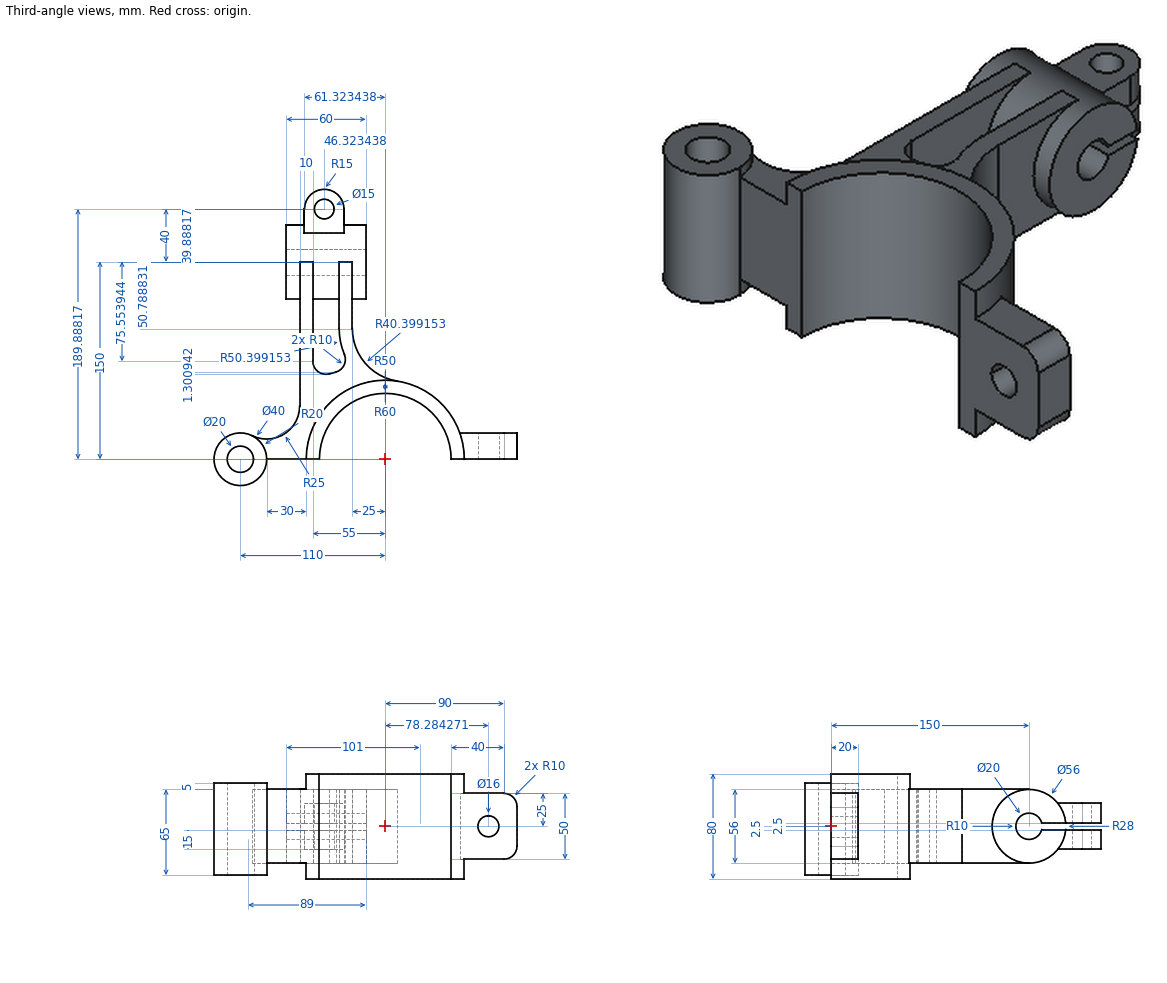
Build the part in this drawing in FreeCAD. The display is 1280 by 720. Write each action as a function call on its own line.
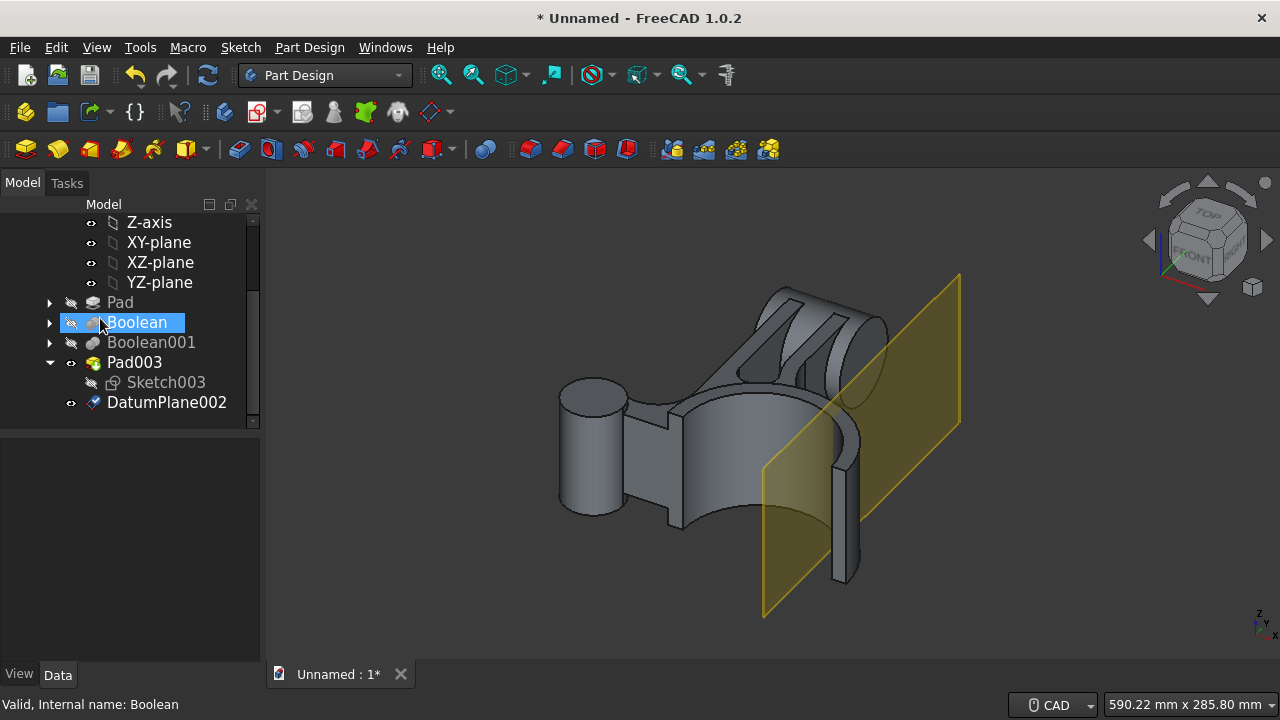
click(116, 403)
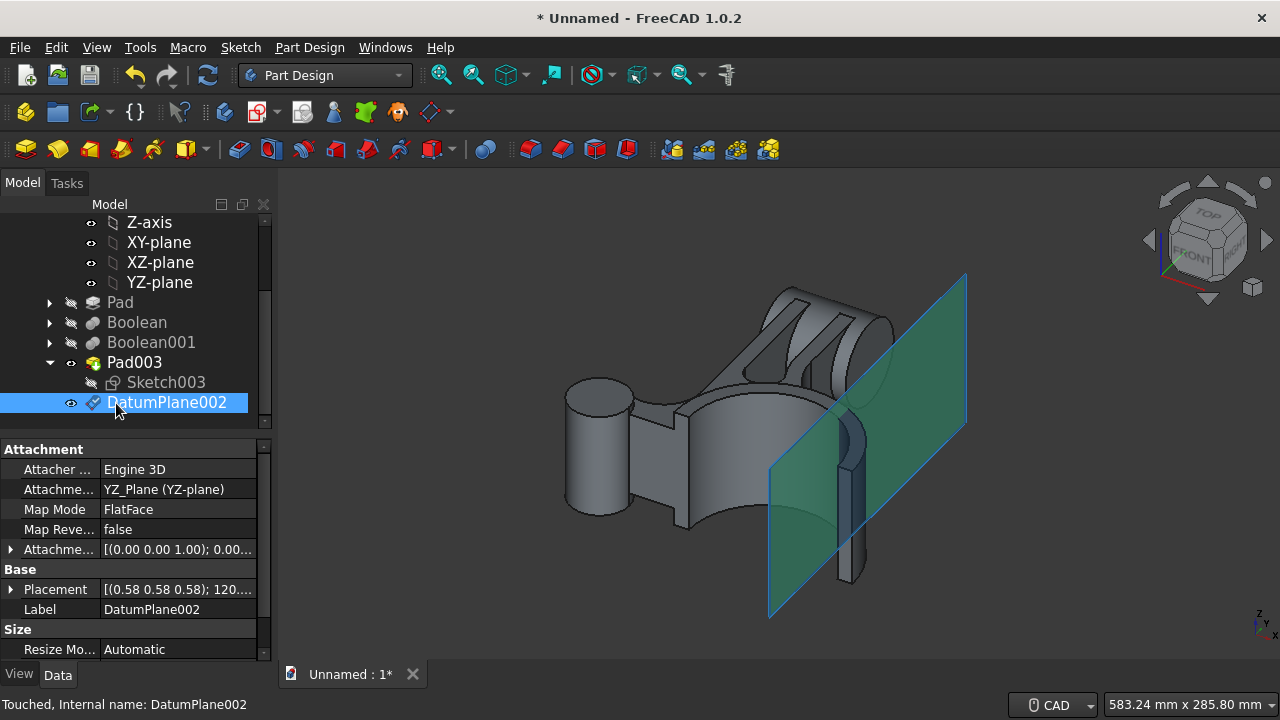
click(258, 112)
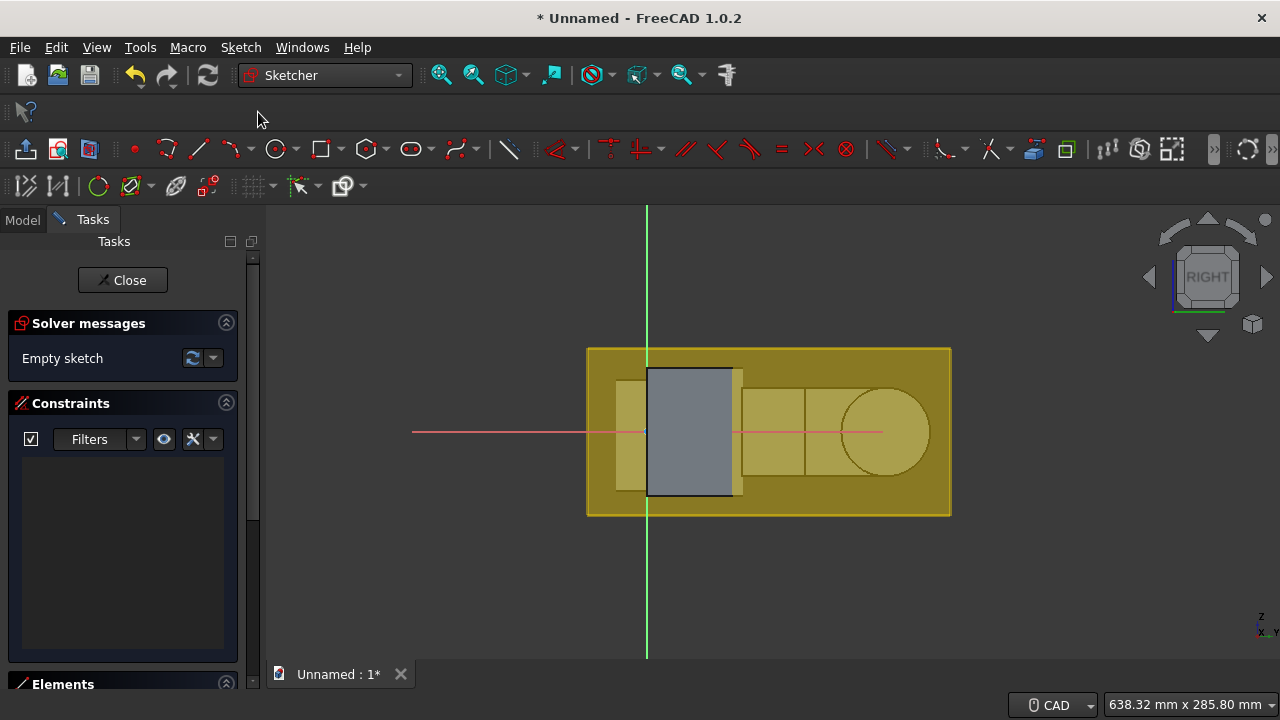
click(90, 150)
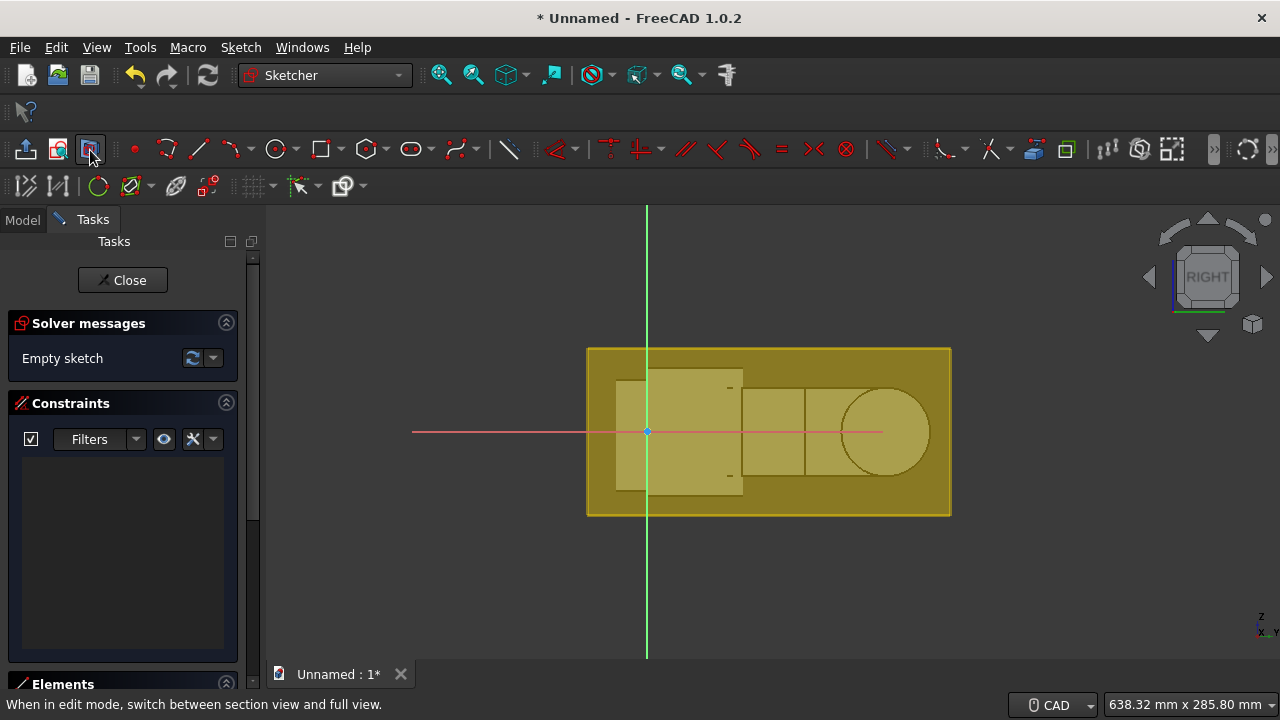
scroll(924, 432, up, 11)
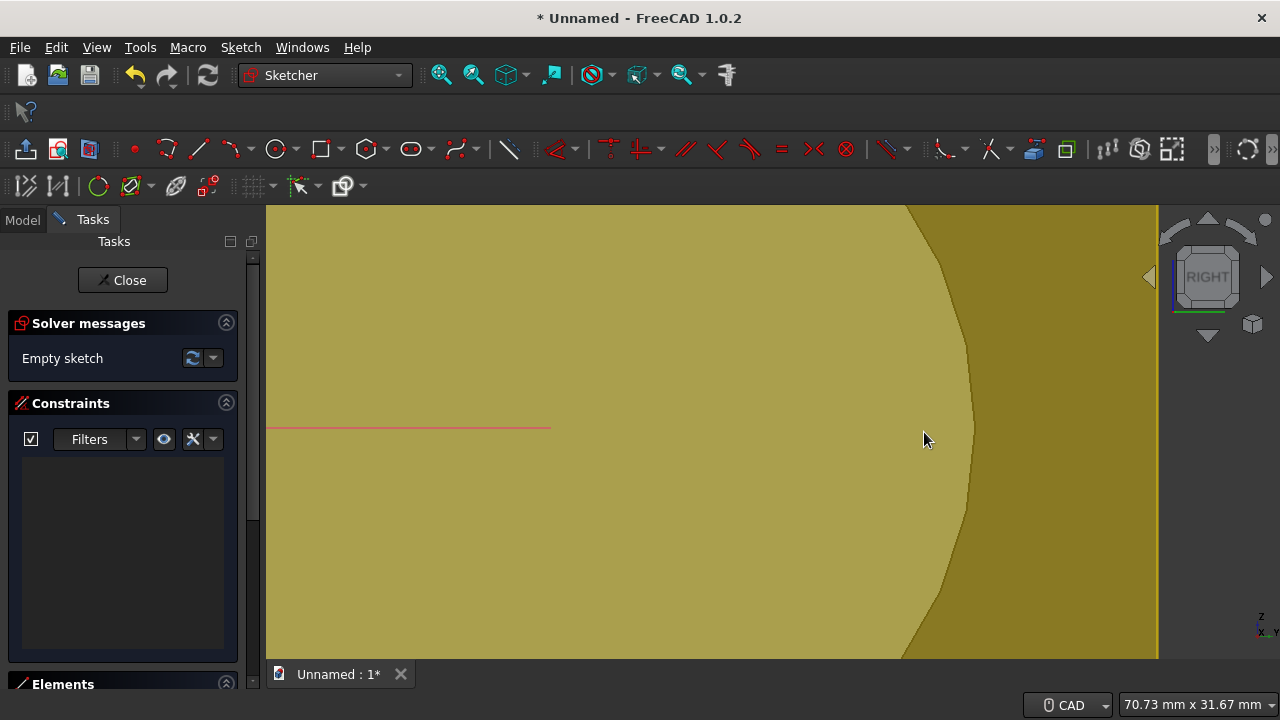
click(200, 150)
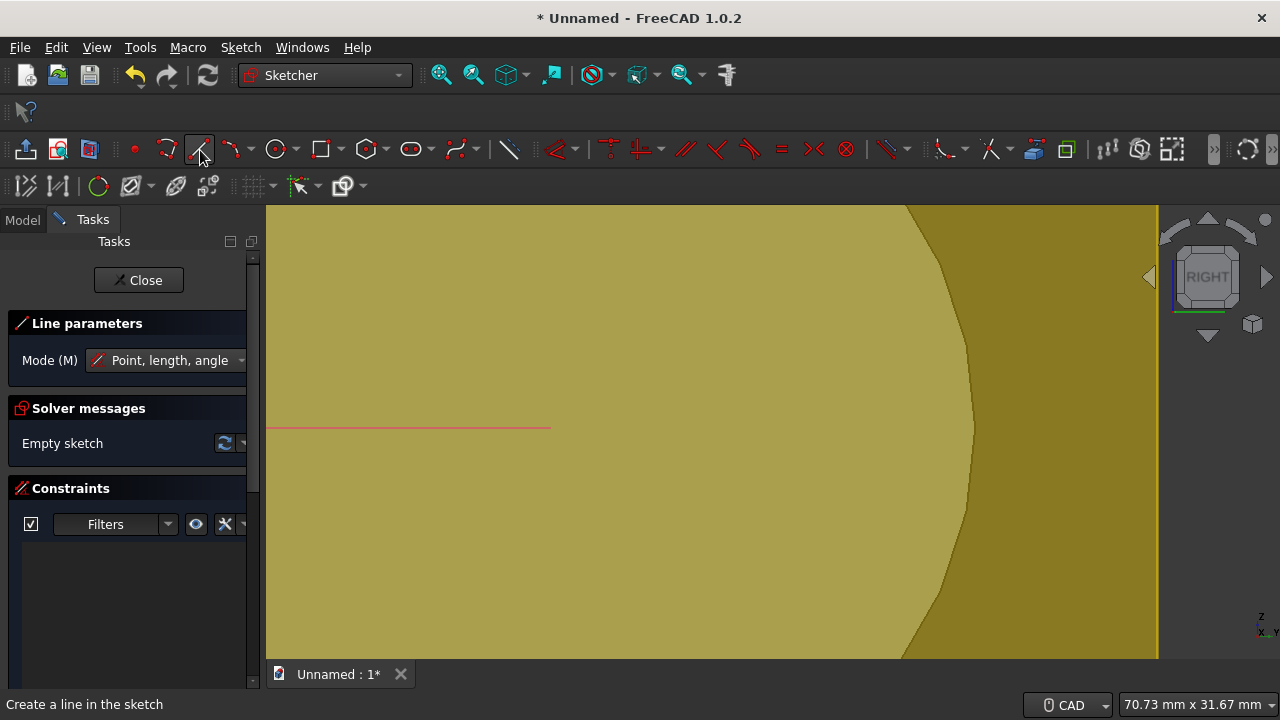
click(713, 392)
click(974, 392)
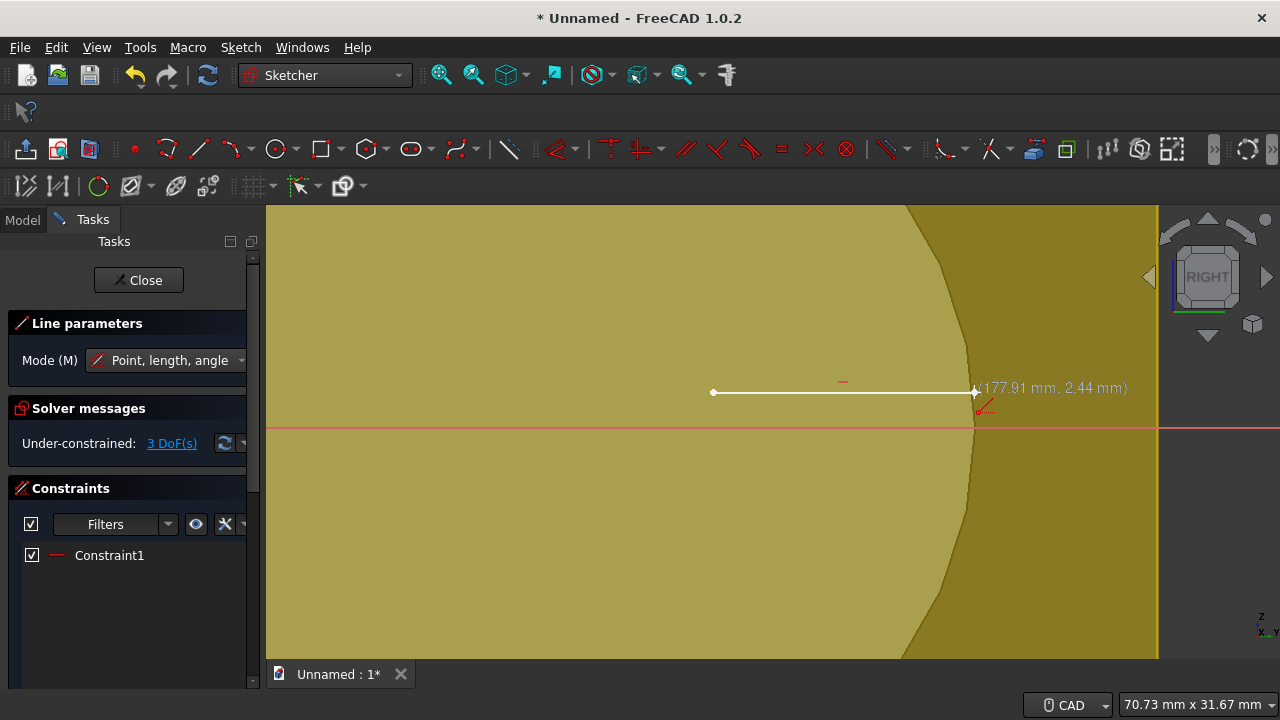
click(974, 464)
click(713, 464)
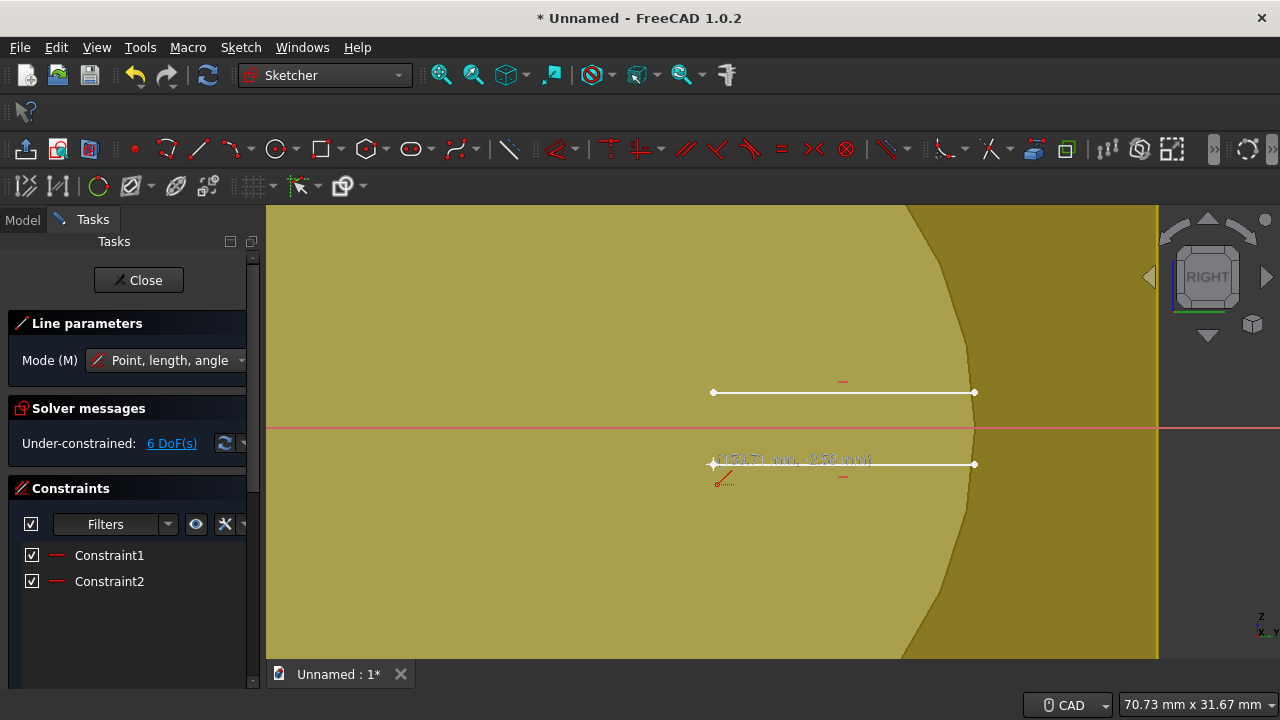
click(232, 150)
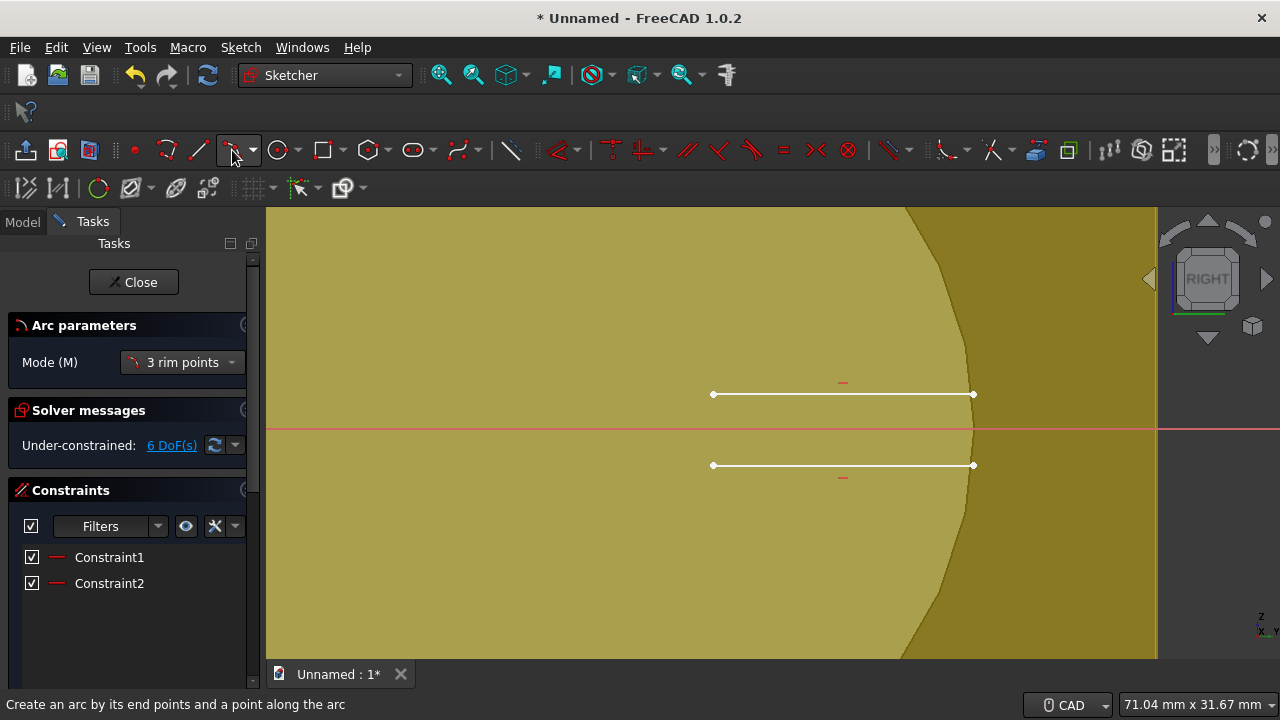
click(973, 394)
click(973, 466)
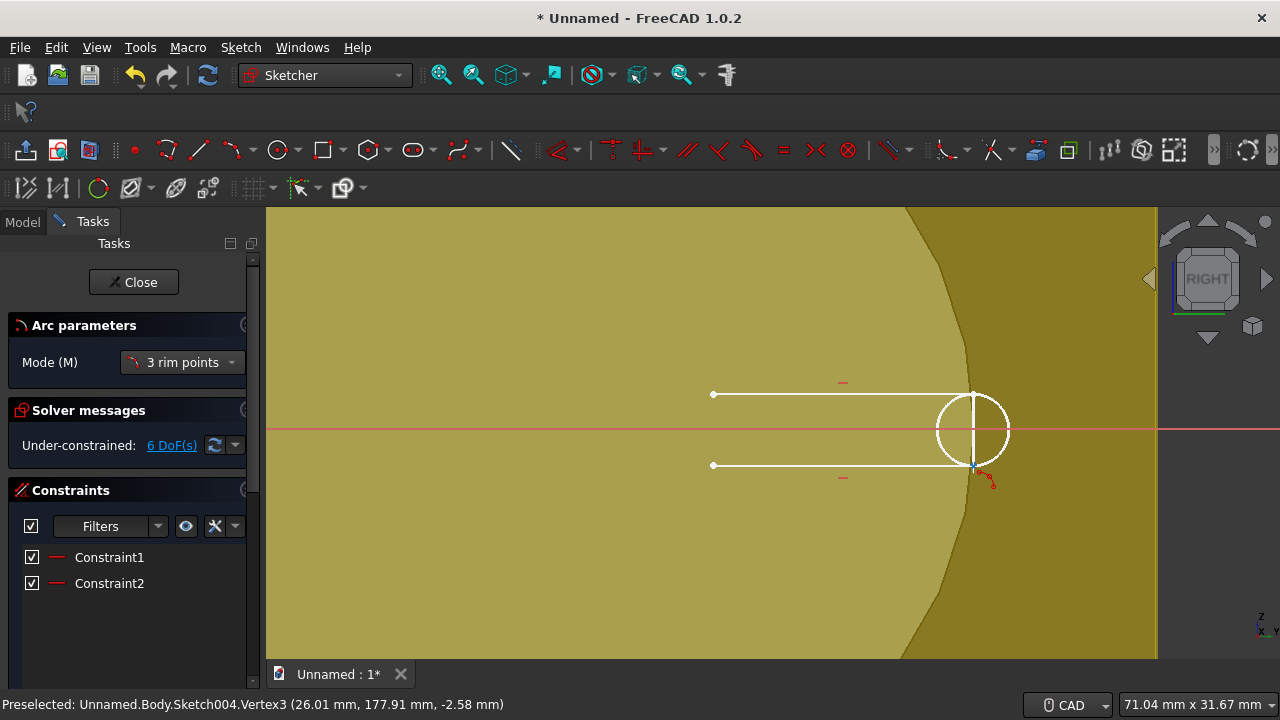
scroll(974, 436, up, 12)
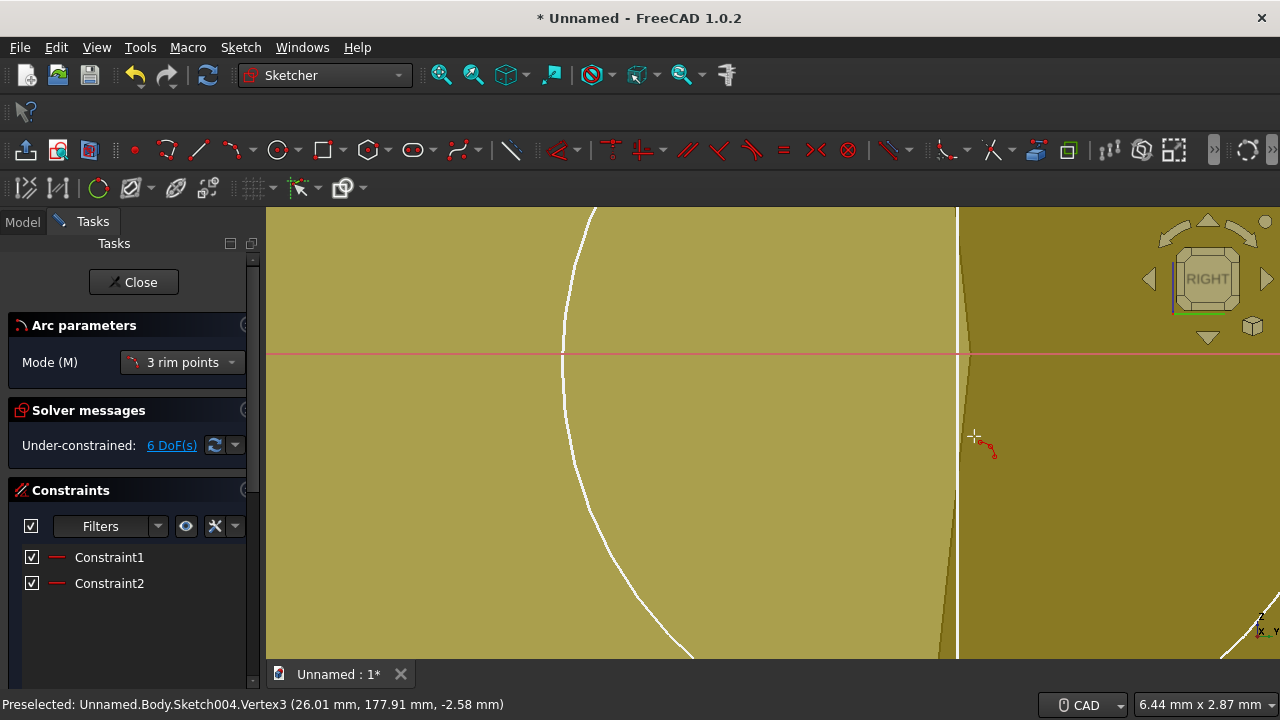
click(970, 432)